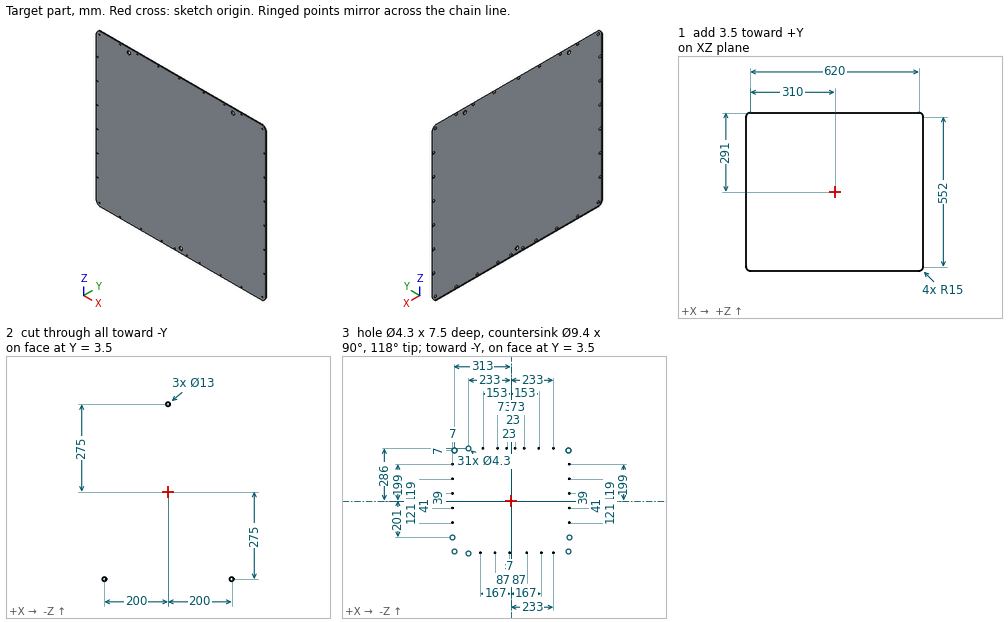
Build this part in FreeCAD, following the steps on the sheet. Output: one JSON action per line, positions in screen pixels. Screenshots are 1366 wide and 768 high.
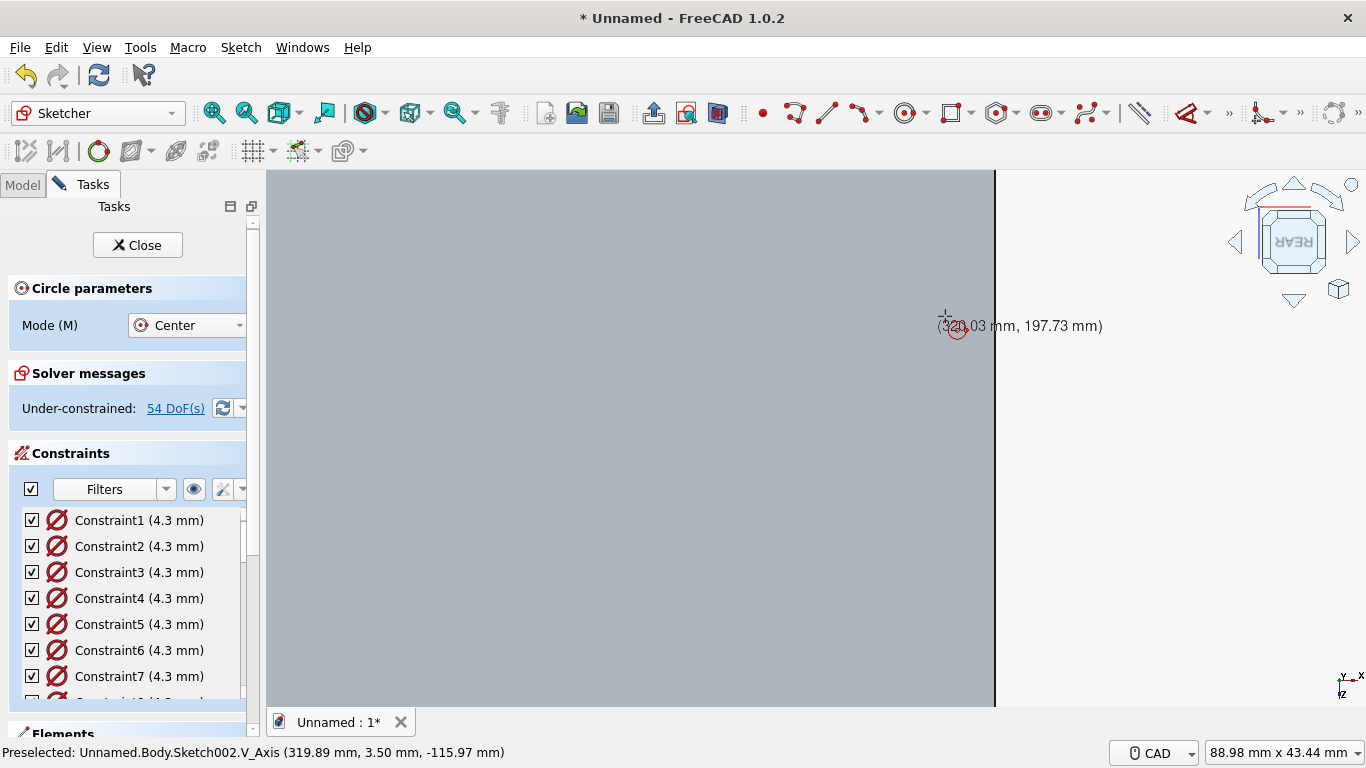
{"action": "scroll", "coordinate": [945, 316], "scroll_direction": "down", "scroll_amount": 15}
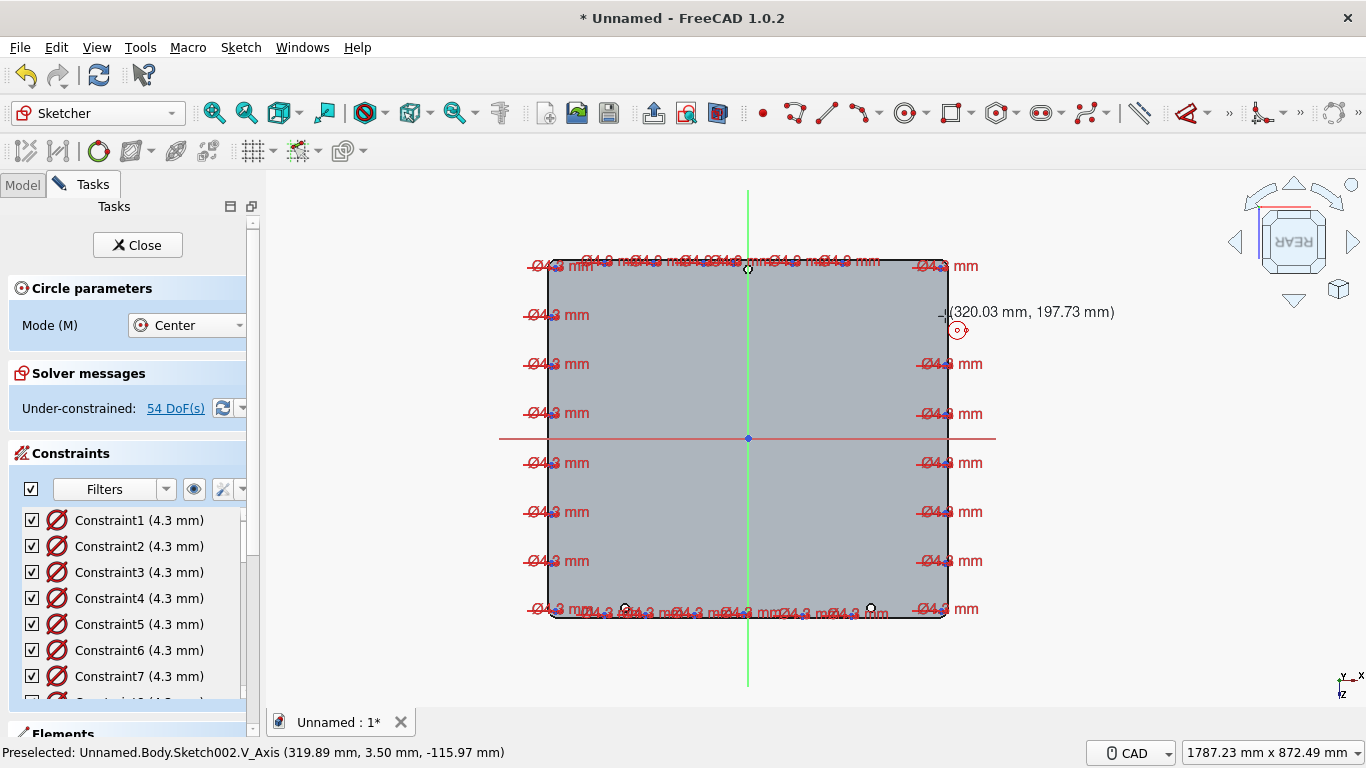
{"action": "left_click", "coordinate": [945, 316]}
{"action": "mouse_move", "coordinate": [946, 315]}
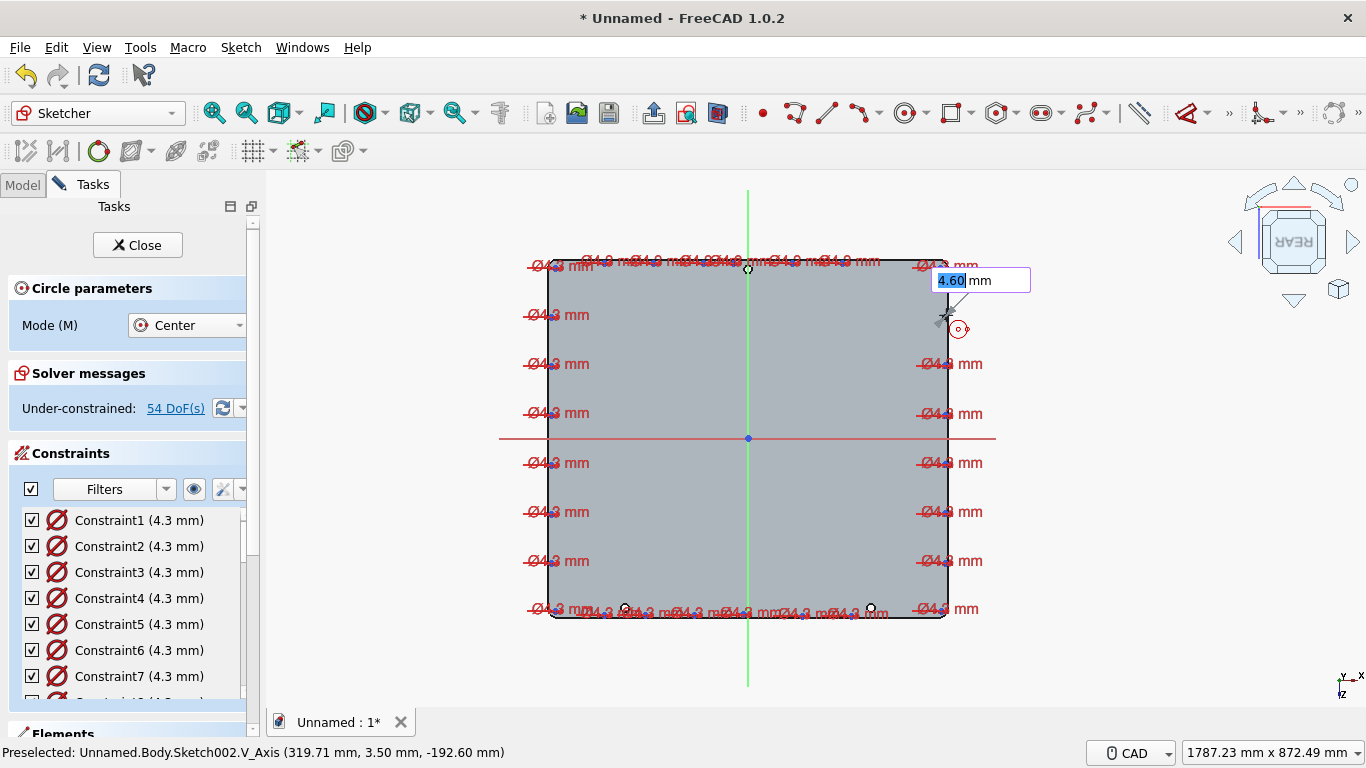
{"action": "type", "text": "4.3"}
{"action": "key", "text": "Return"}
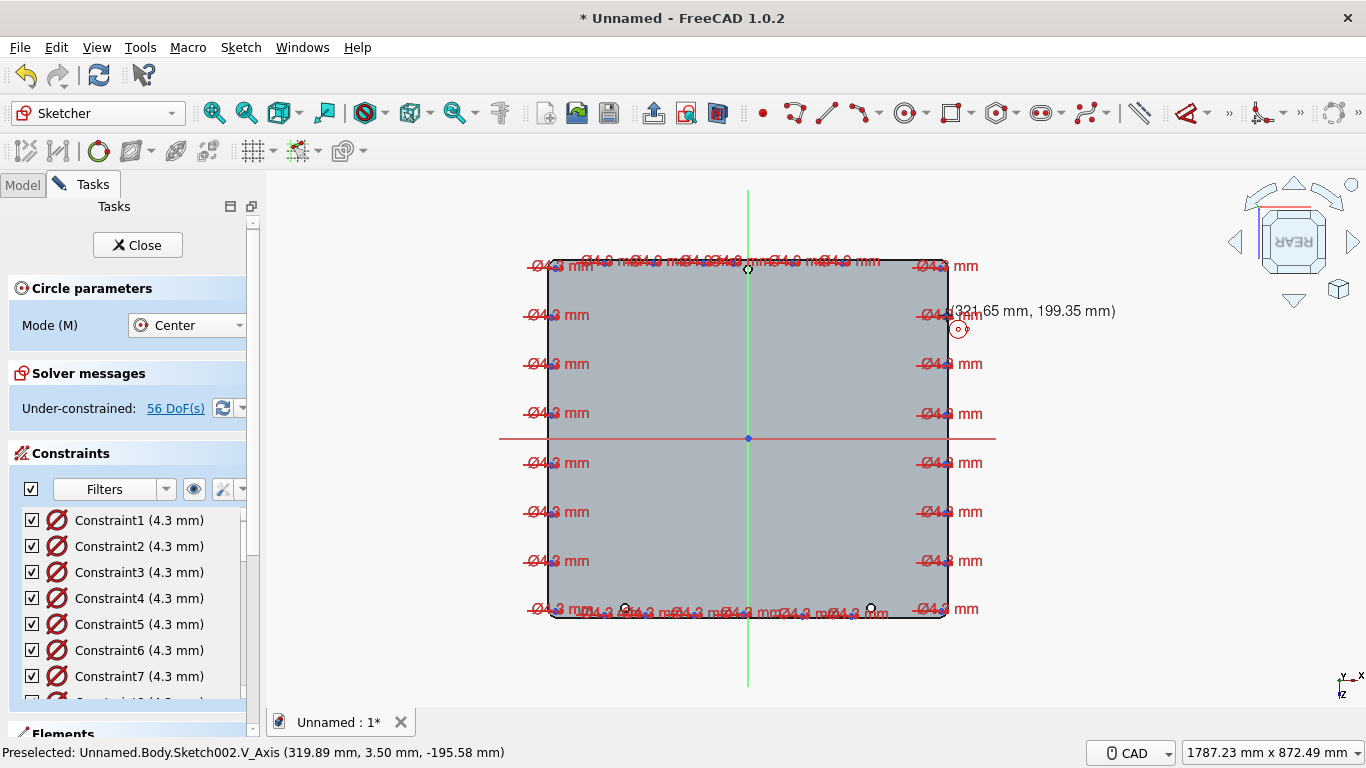
{"action": "scroll", "coordinate": [891, 263], "scroll_direction": "up", "scroll_amount": 15}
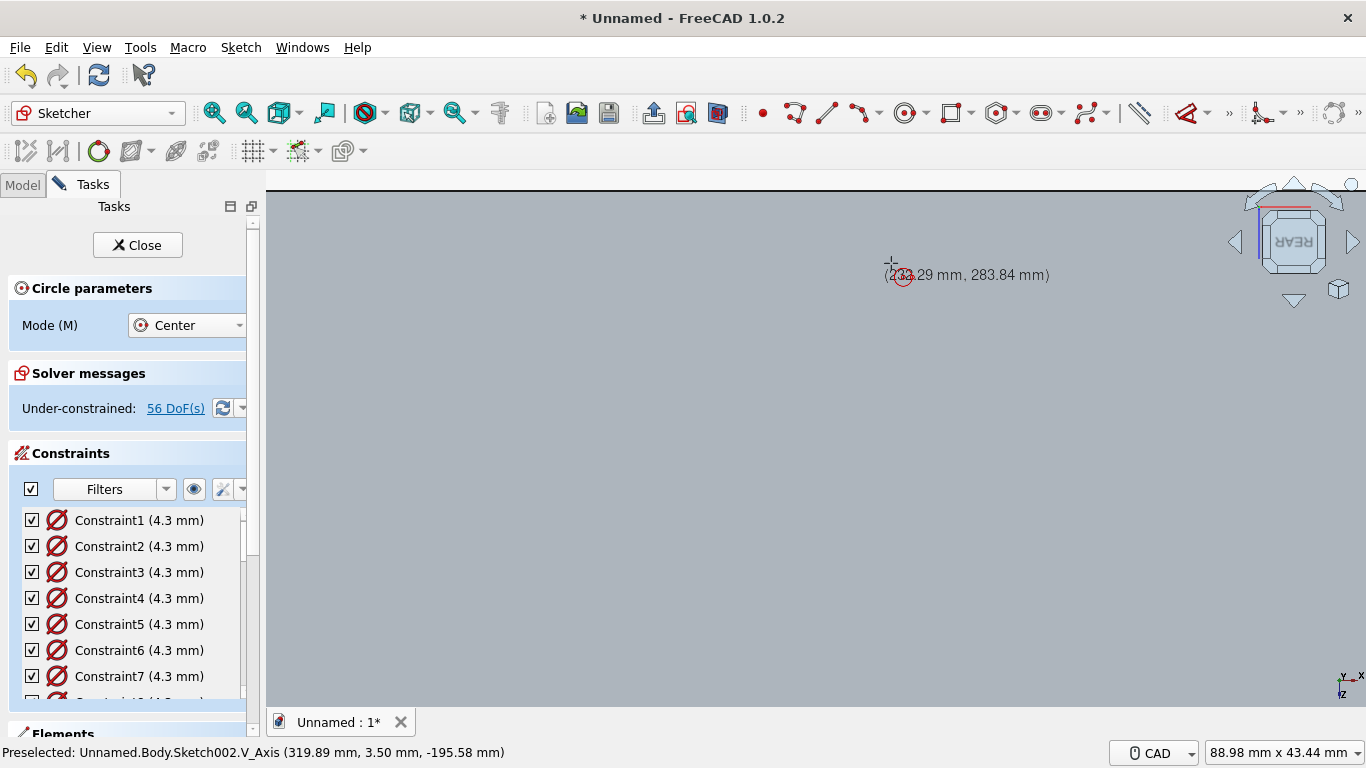
{"action": "scroll", "coordinate": [891, 263], "scroll_direction": "down", "scroll_amount": 15}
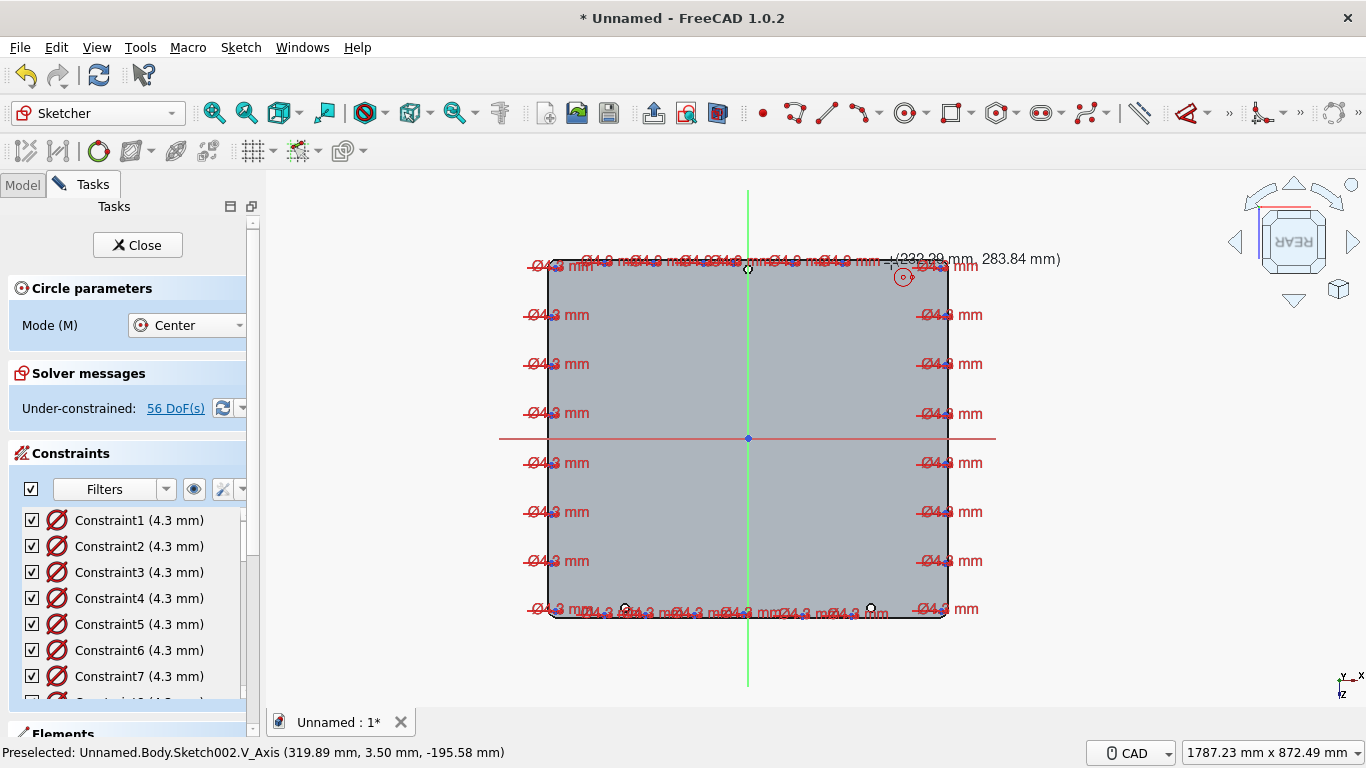
{"action": "left_click", "coordinate": [891, 263]}
{"action": "mouse_move", "coordinate": [892, 262]}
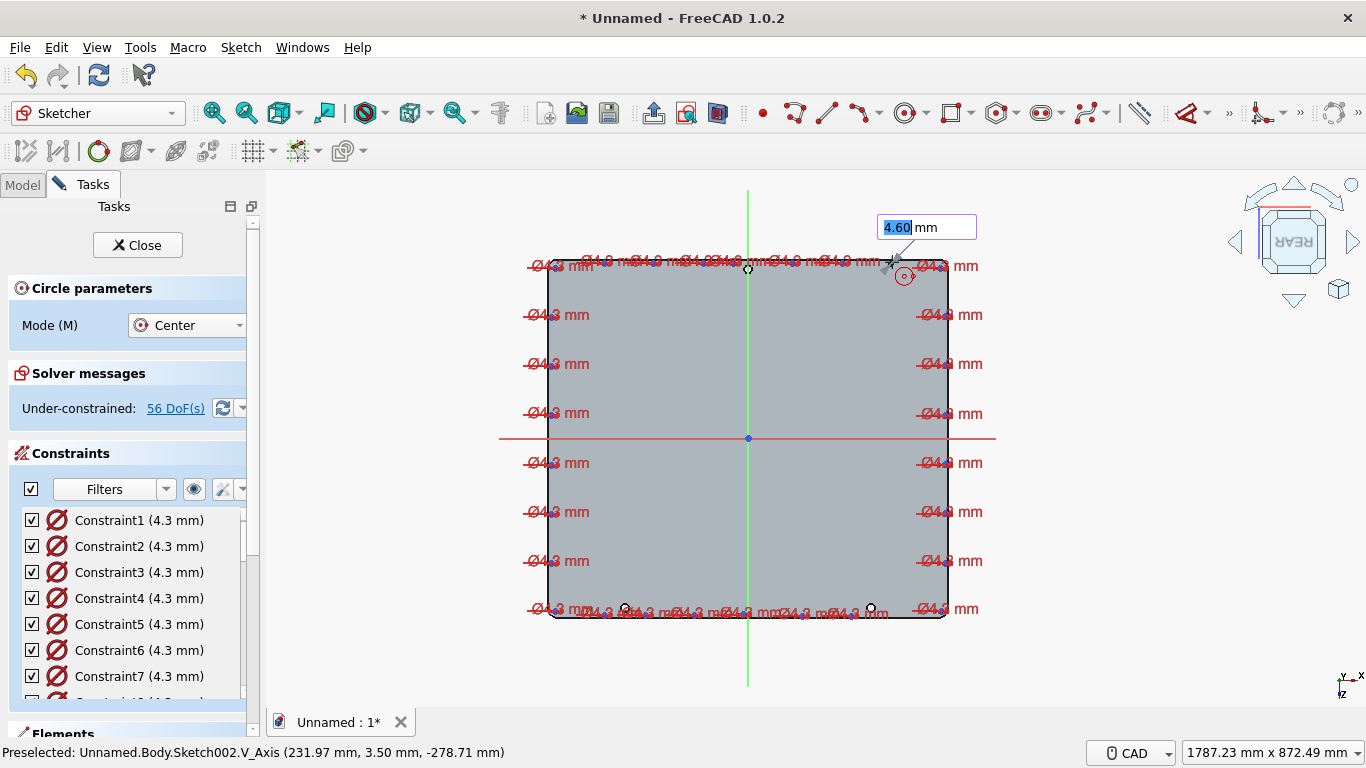
{"action": "type", "text": "4.3"}
{"action": "key", "text": "Return"}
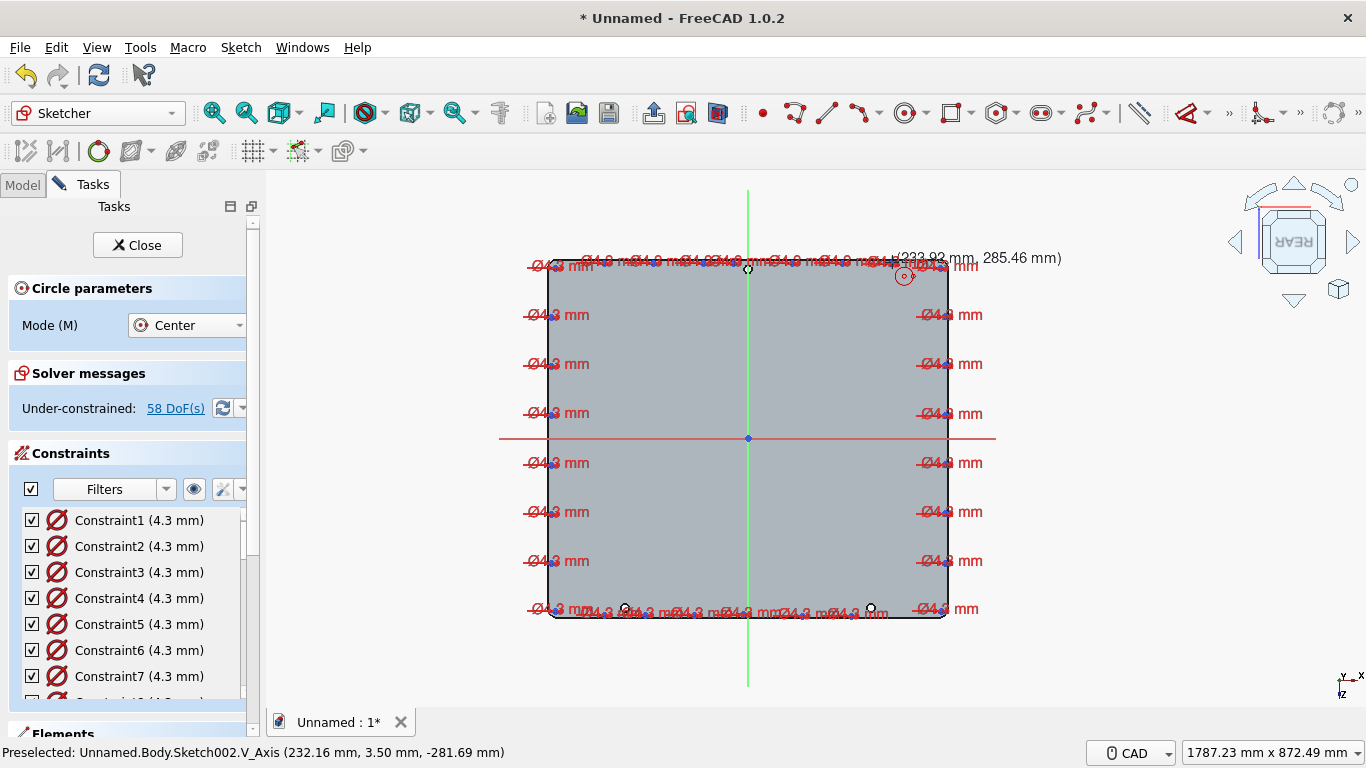
{"action": "scroll", "coordinate": [762, 263], "scroll_direction": "up", "scroll_amount": 15}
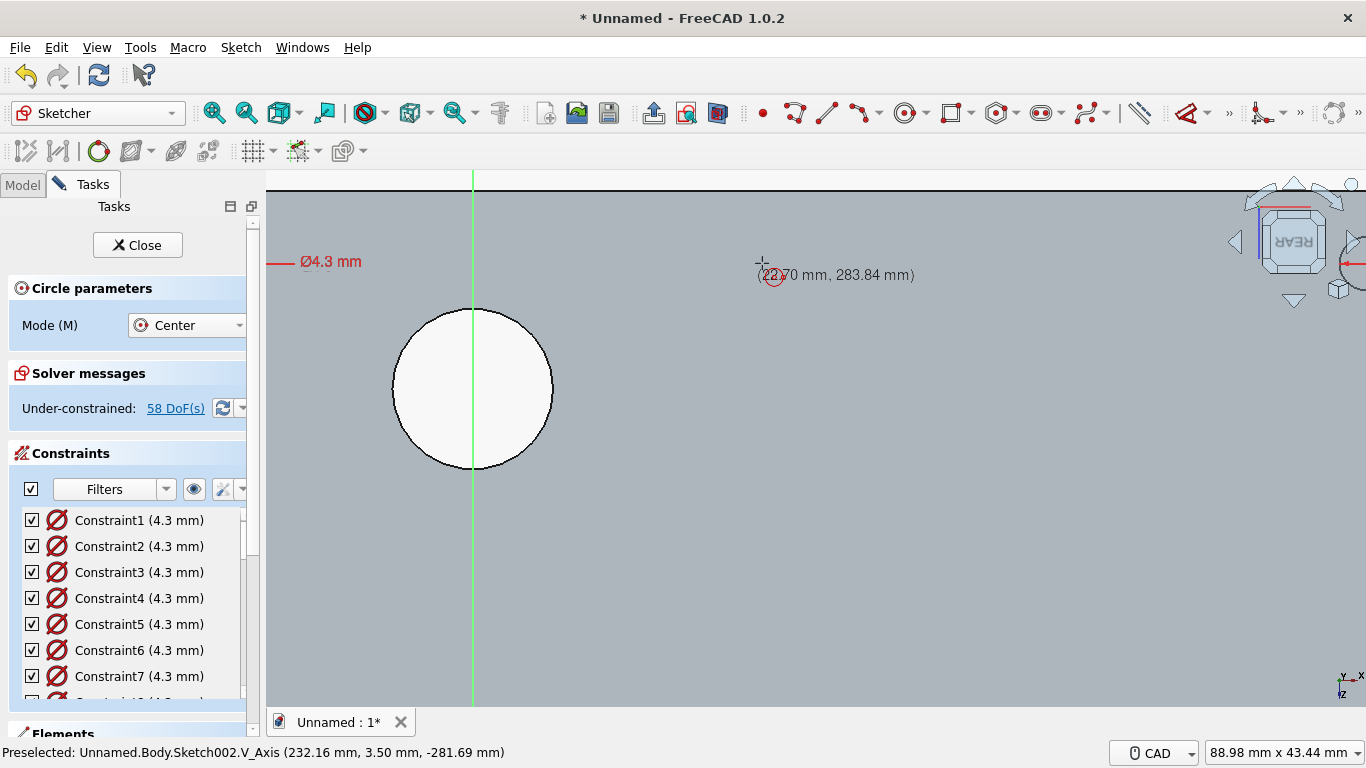
{"action": "scroll", "coordinate": [762, 263], "scroll_direction": "down", "scroll_amount": 15}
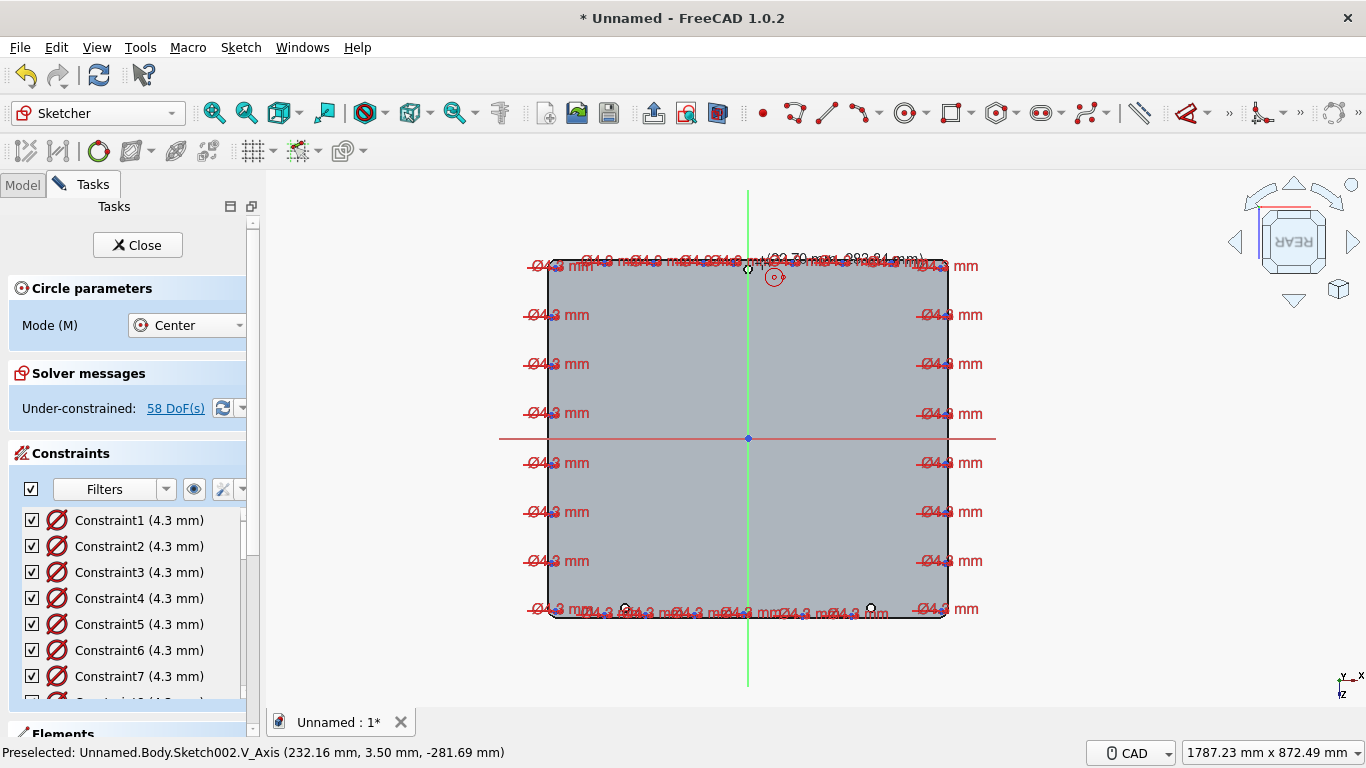
{"action": "left_click", "coordinate": [762, 263]}
{"action": "mouse_move", "coordinate": [763, 262]}